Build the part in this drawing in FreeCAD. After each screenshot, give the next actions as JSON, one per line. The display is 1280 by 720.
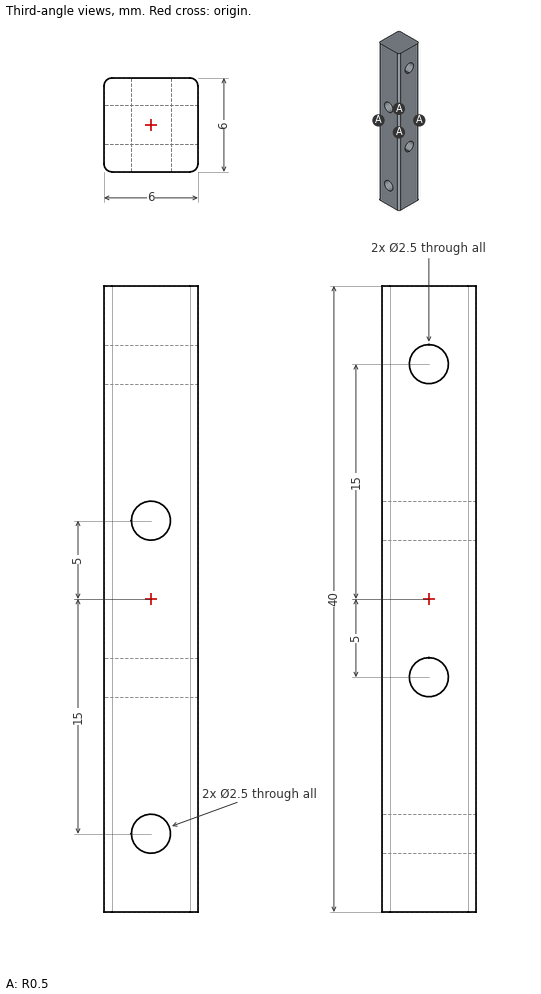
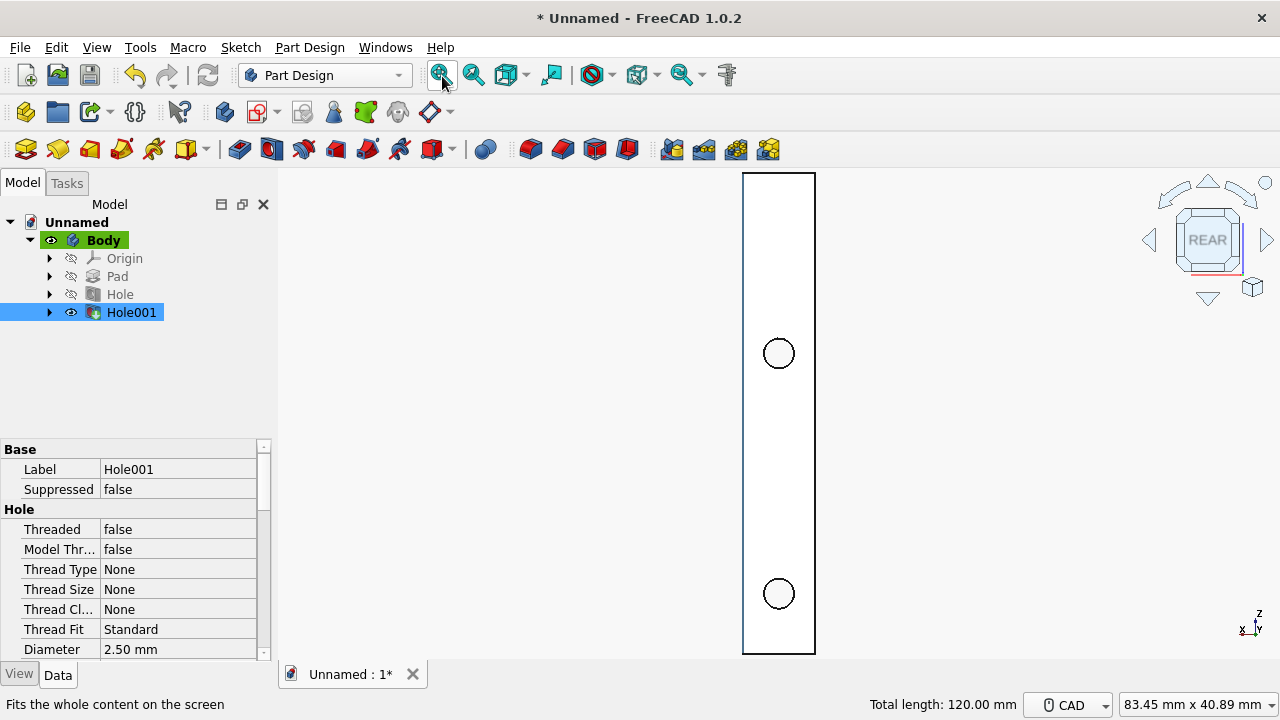
{"action": "left_click", "coordinate": [815, 413], "text": "ctrl"}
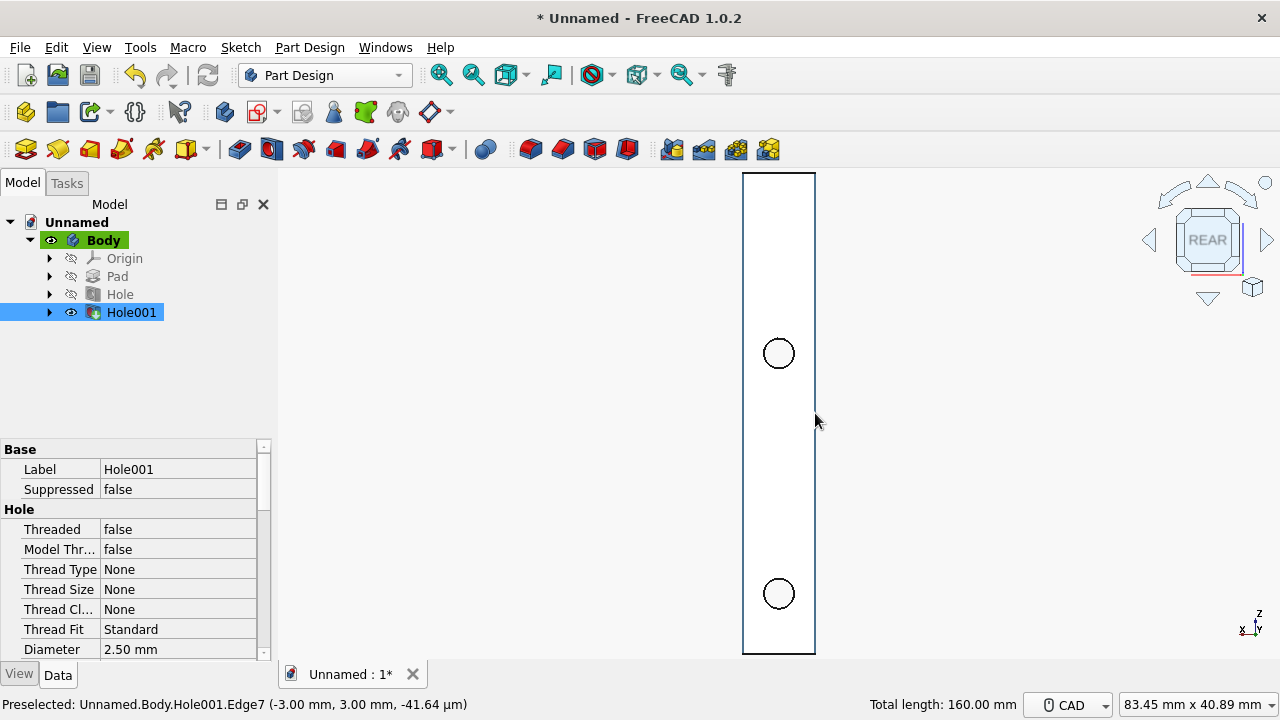
{"action": "left_click", "coordinate": [532, 150]}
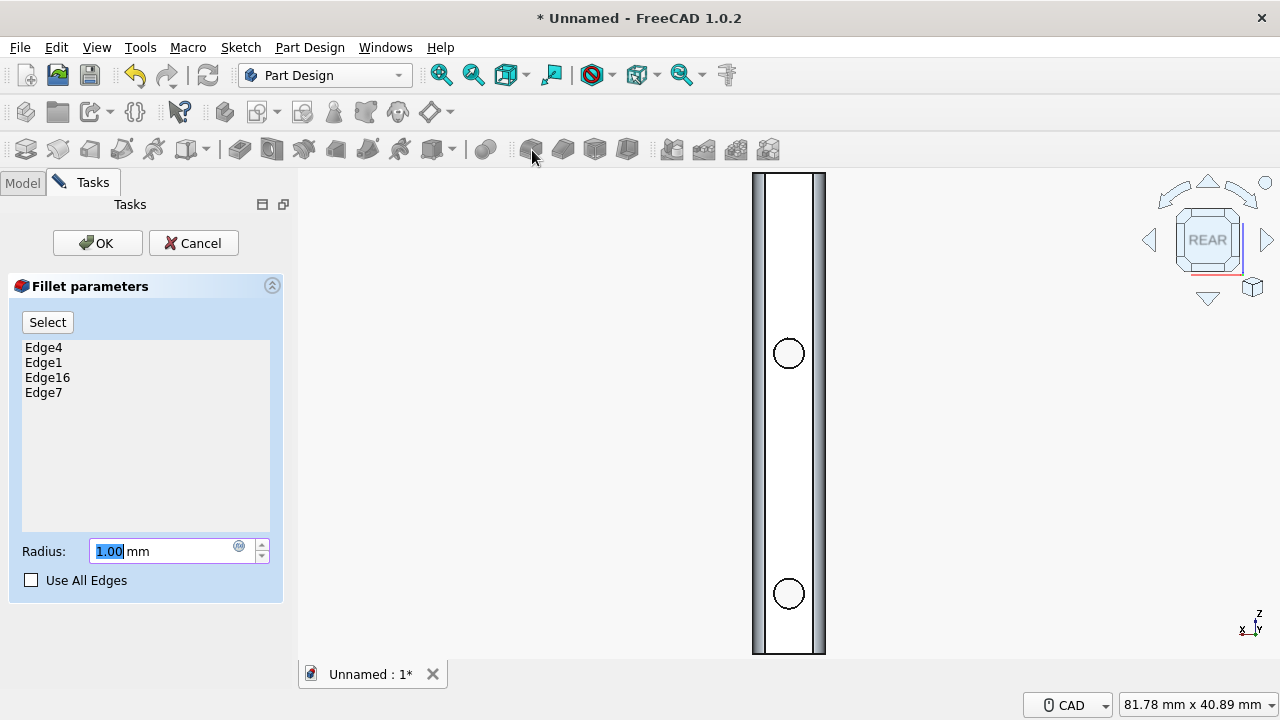
{"action": "type", "text": "0.5"}
{"action": "key", "text": "Tab"}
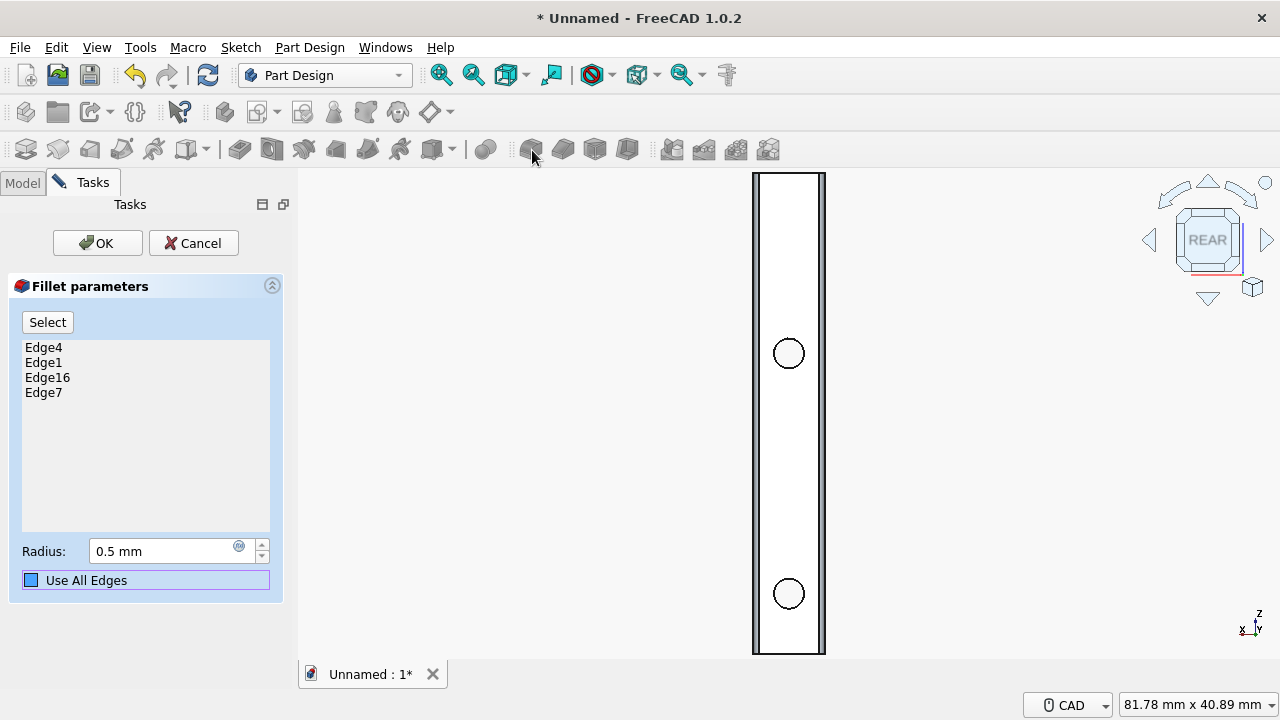
{"action": "left_click", "coordinate": [98, 243]}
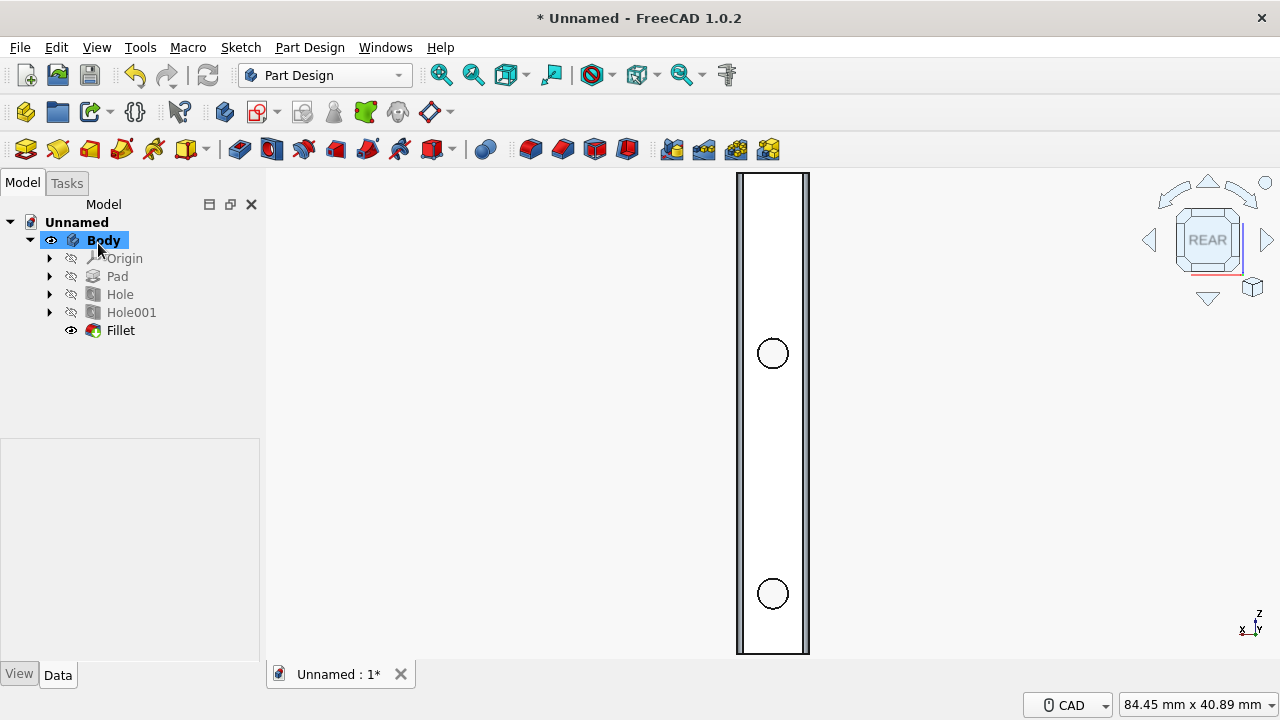
{"action": "key", "text": "0"}